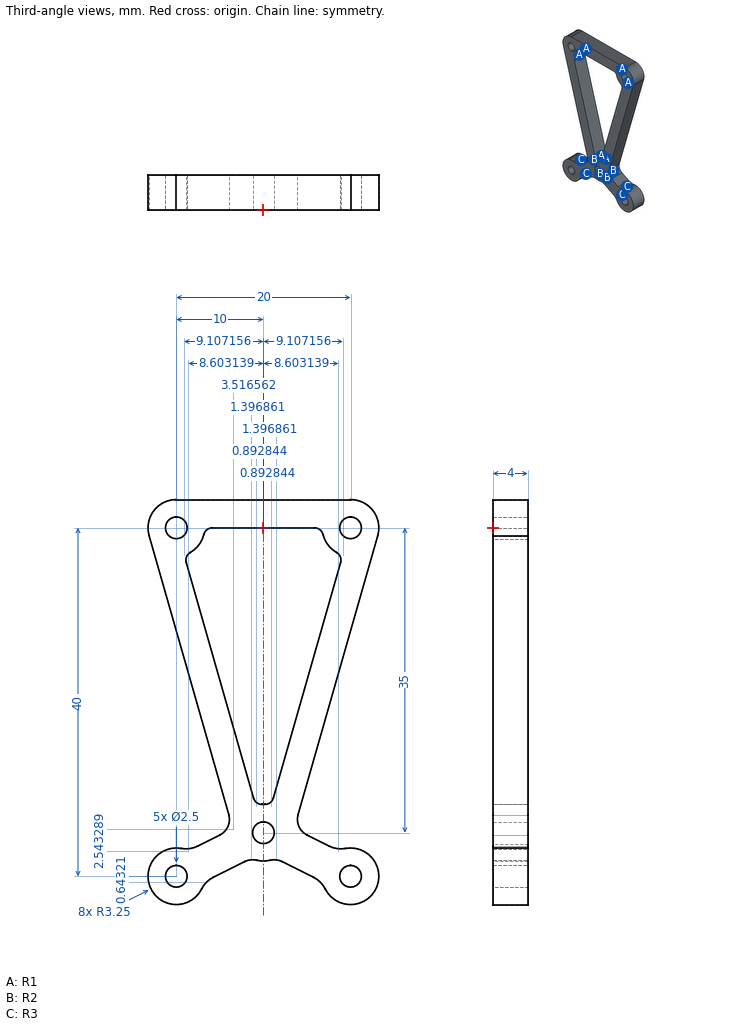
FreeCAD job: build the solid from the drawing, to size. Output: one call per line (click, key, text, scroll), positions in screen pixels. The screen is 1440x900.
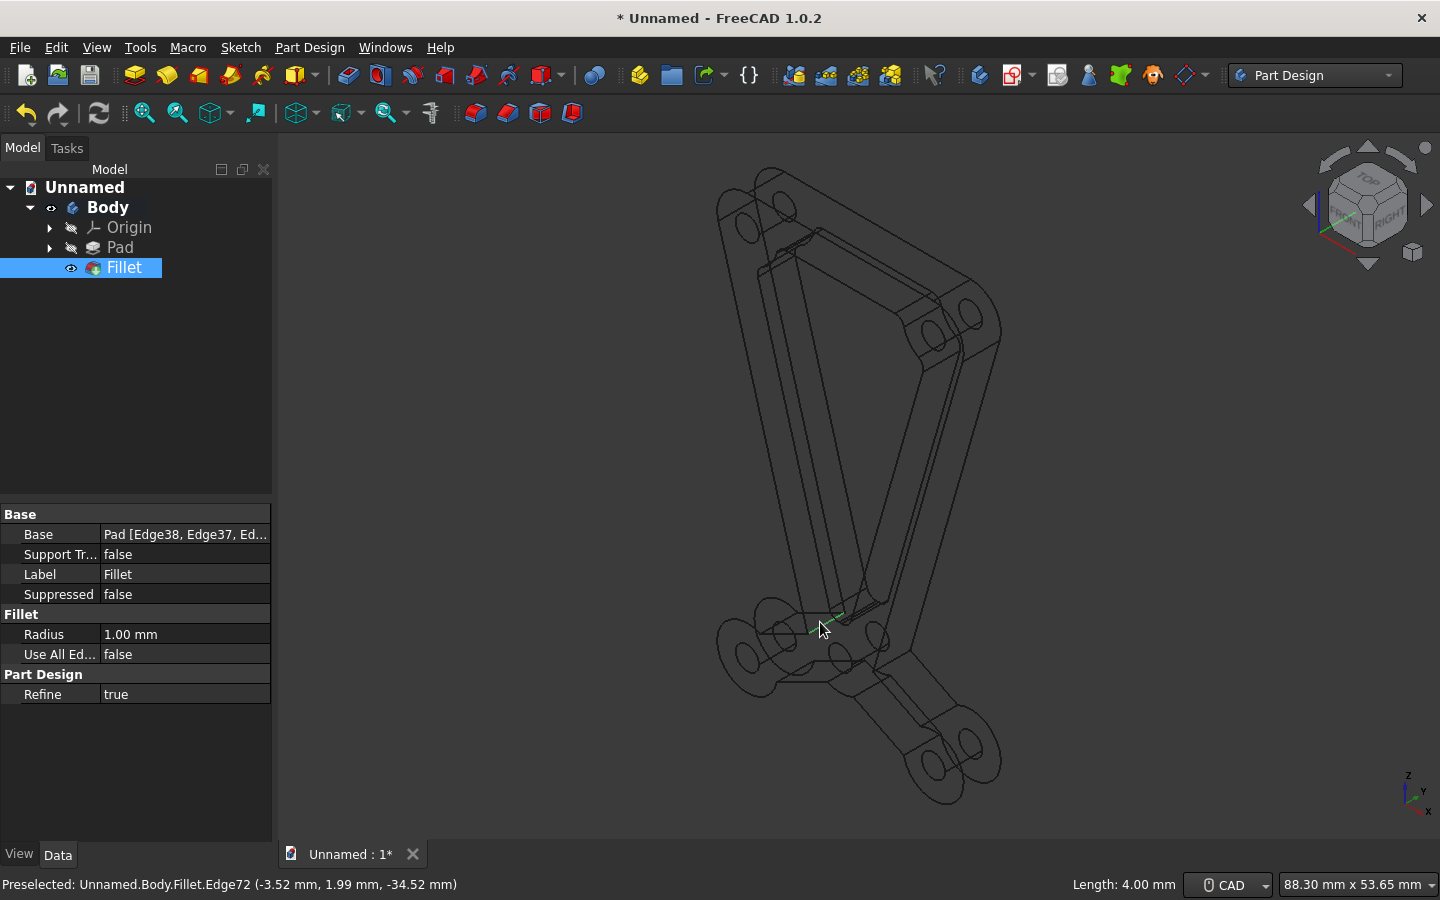
click(835, 677, ctrl)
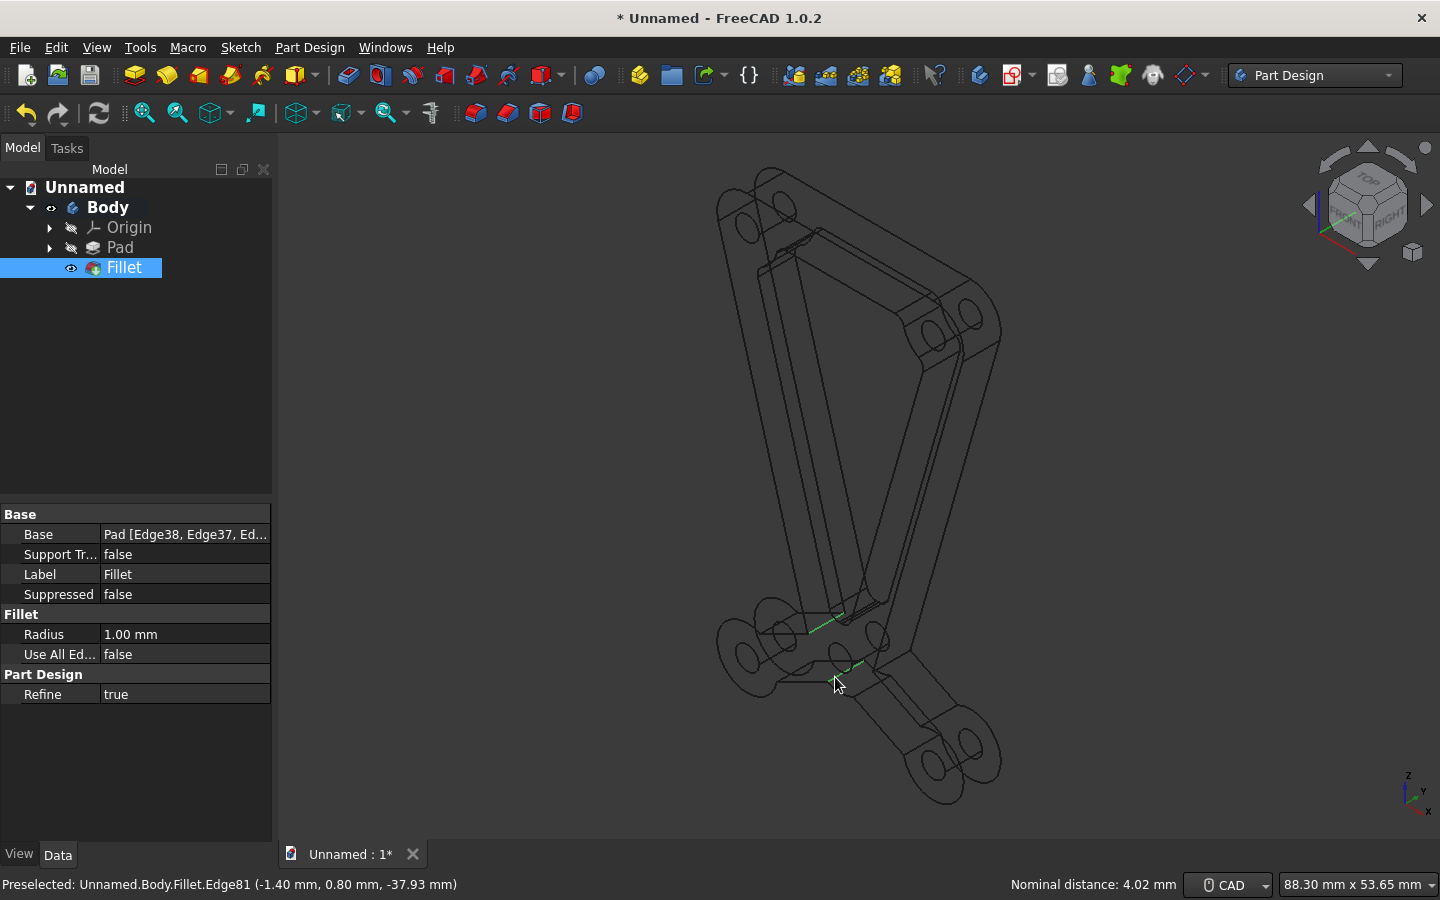
click(872, 685, ctrl)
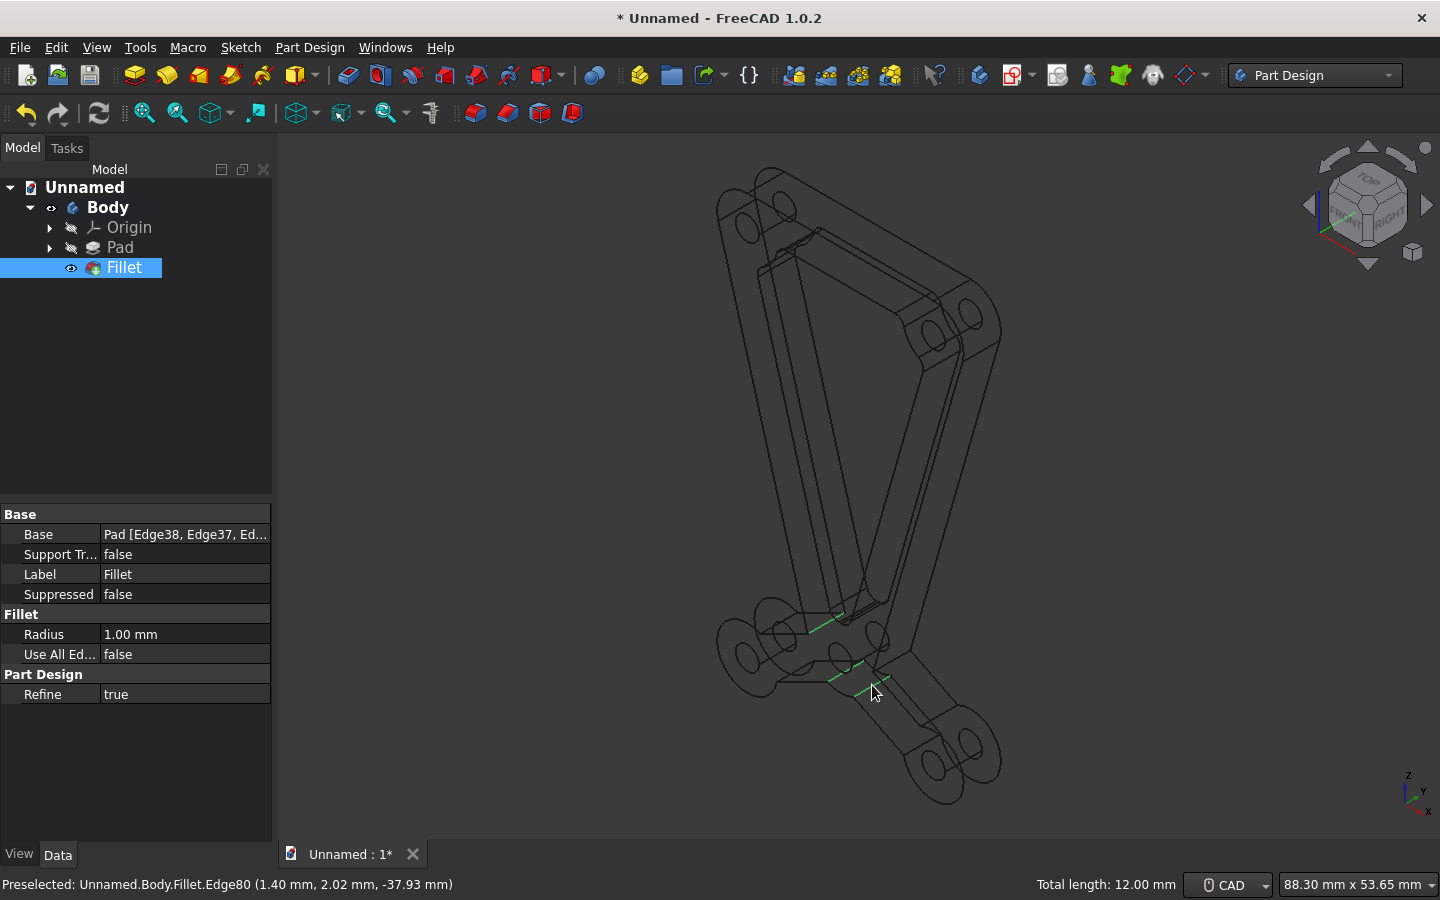
click(892, 660, ctrl)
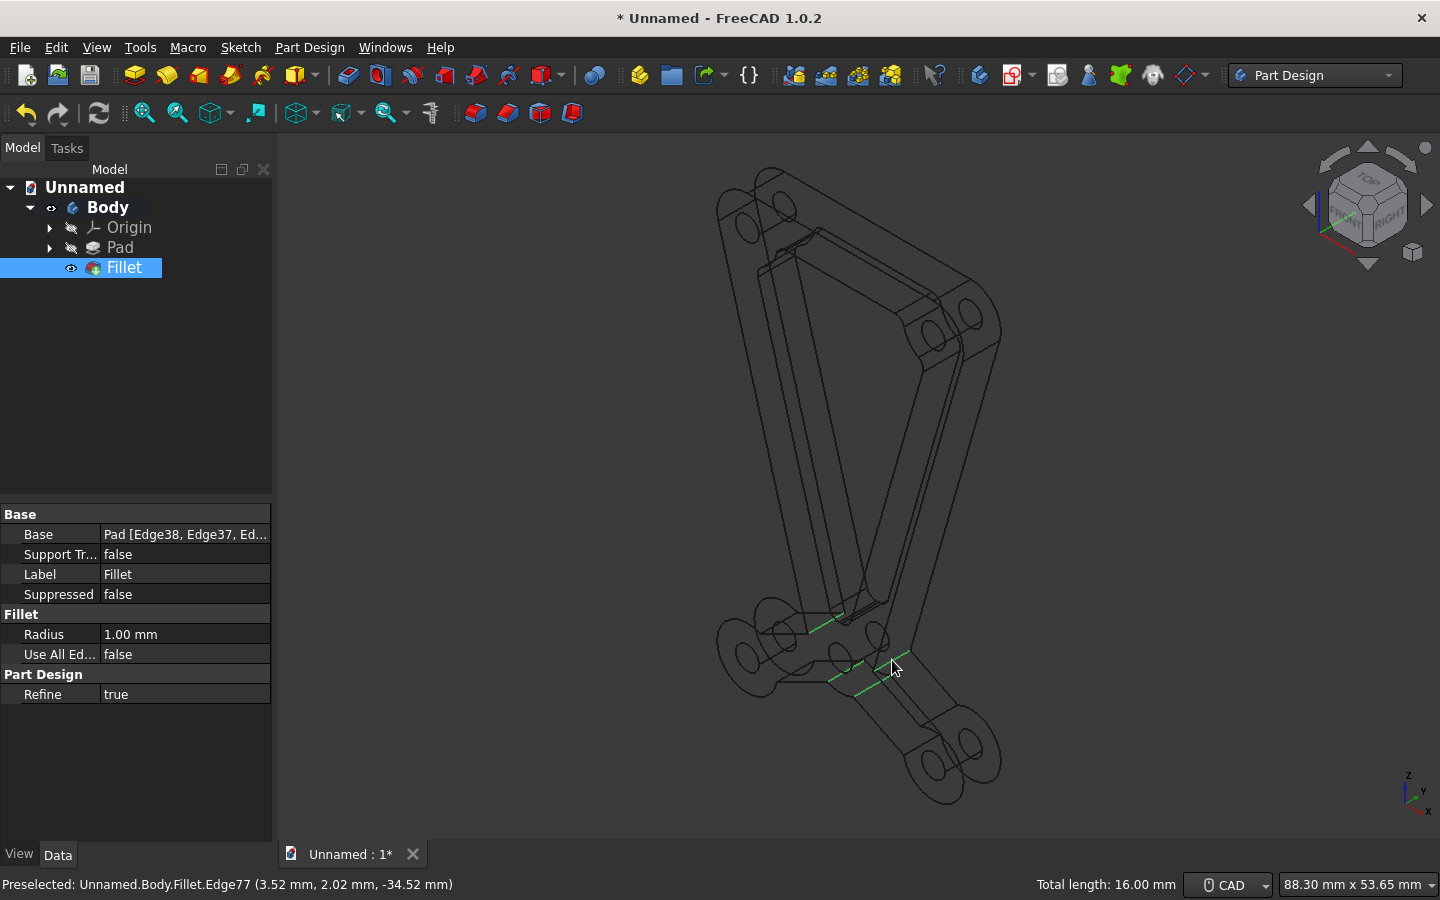
key(v)
key(1)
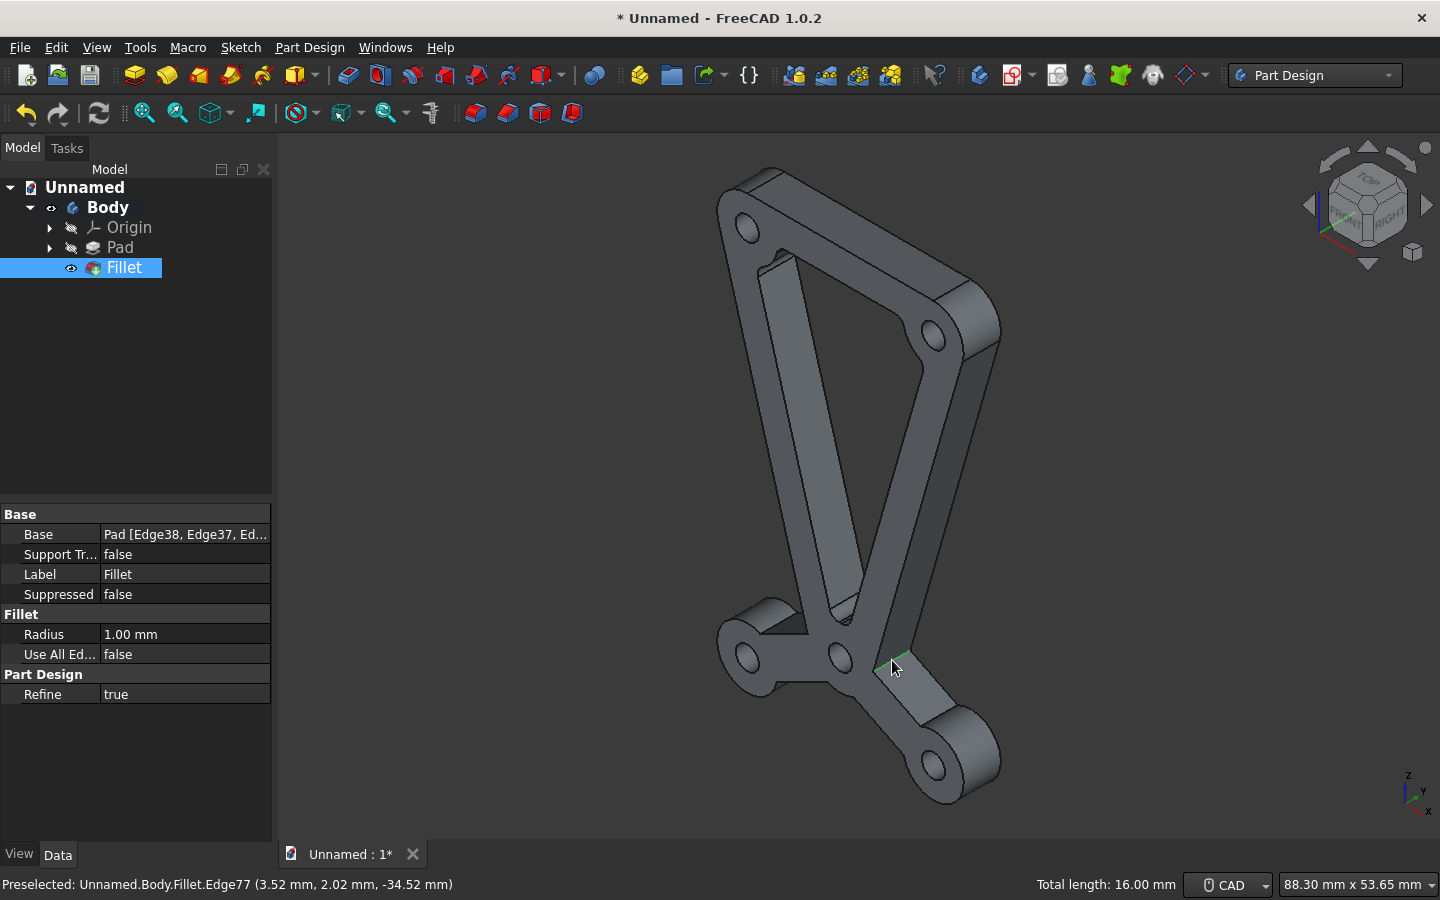
click(476, 114)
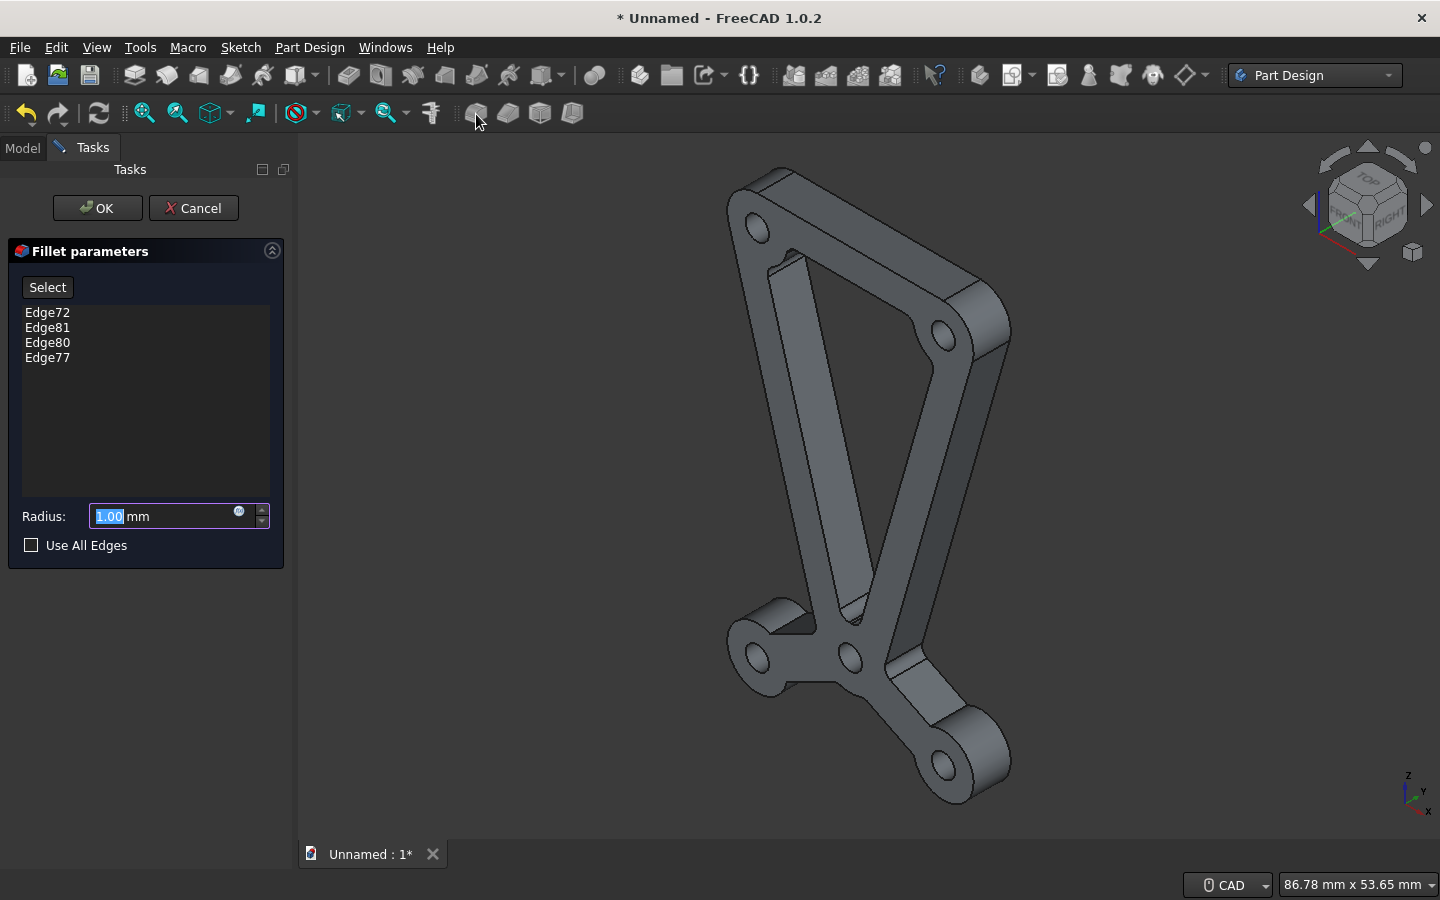
text(2)
key(Tab)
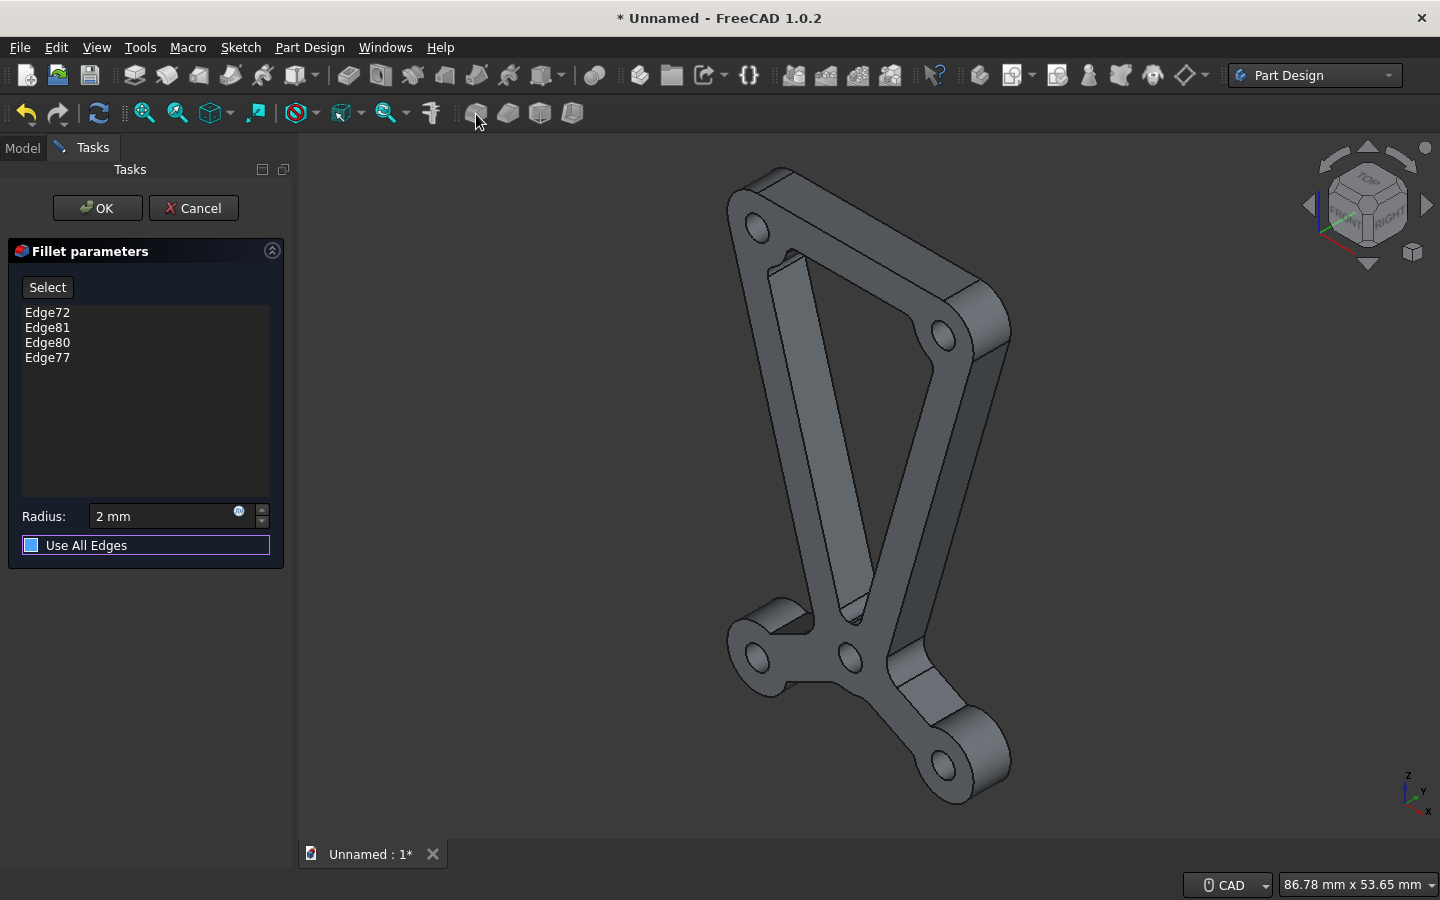
click(98, 208)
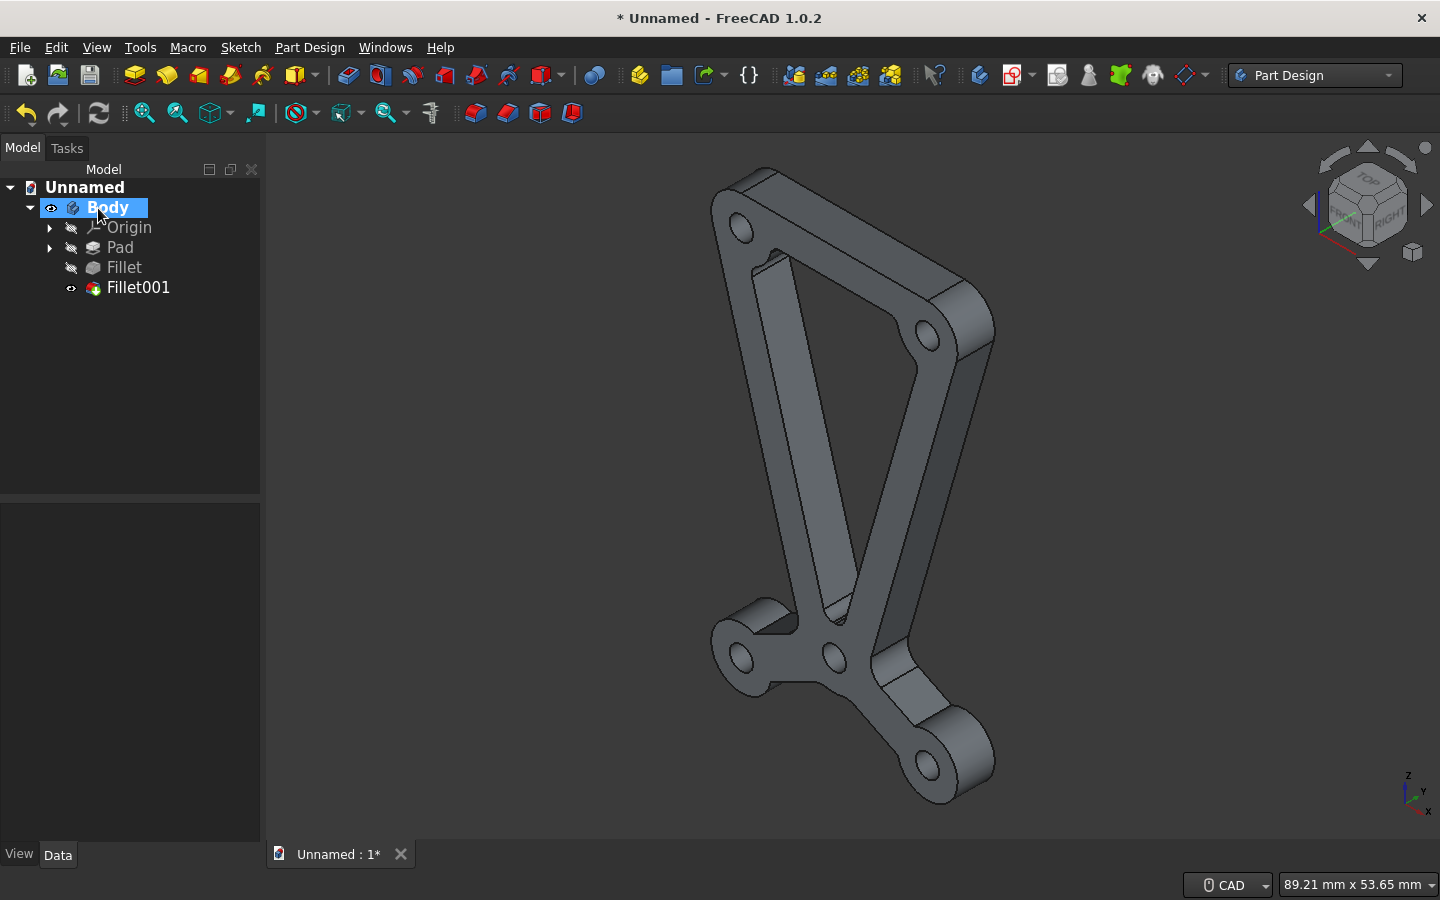
key(2)